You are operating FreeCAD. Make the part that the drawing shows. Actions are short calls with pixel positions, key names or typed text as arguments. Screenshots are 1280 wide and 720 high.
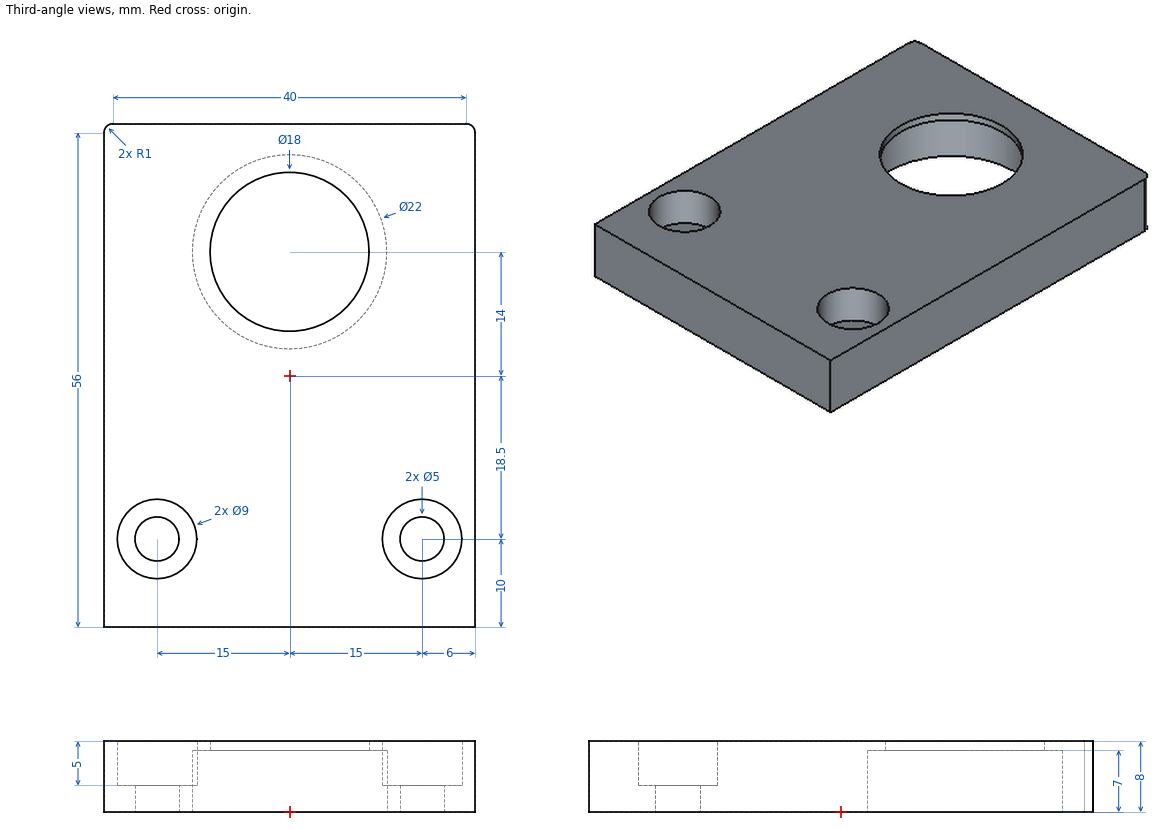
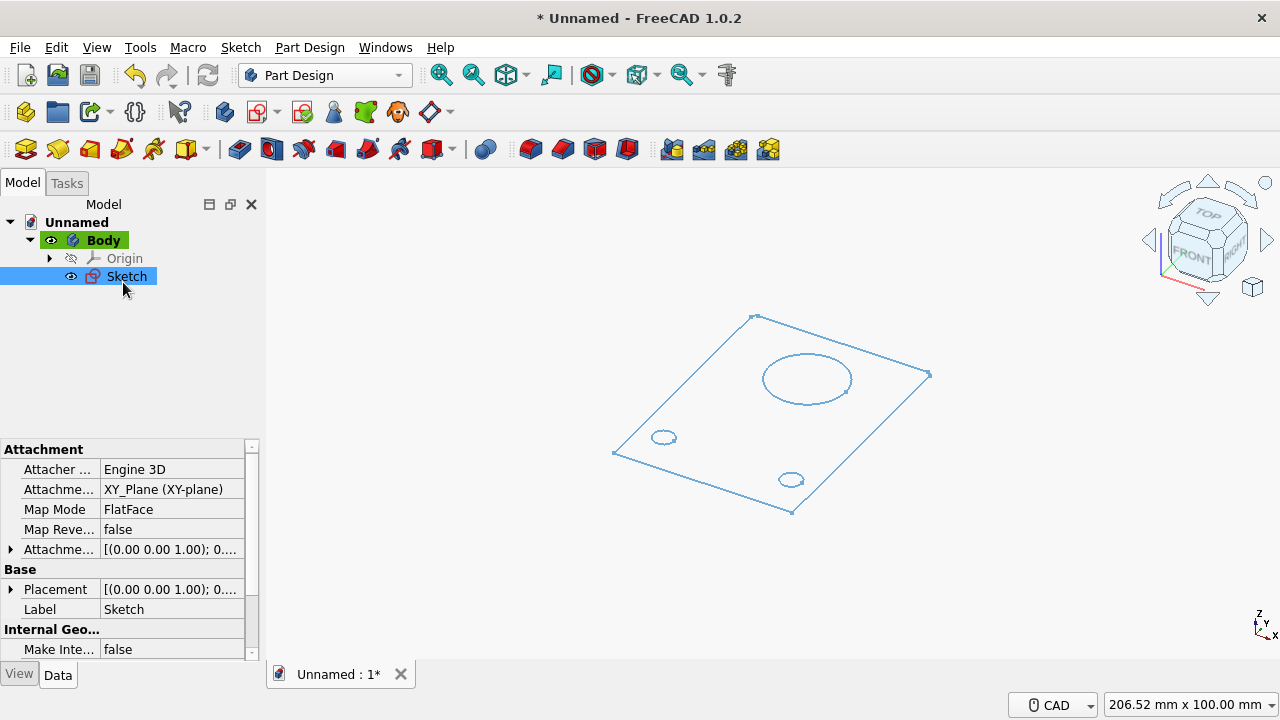
click(26, 150)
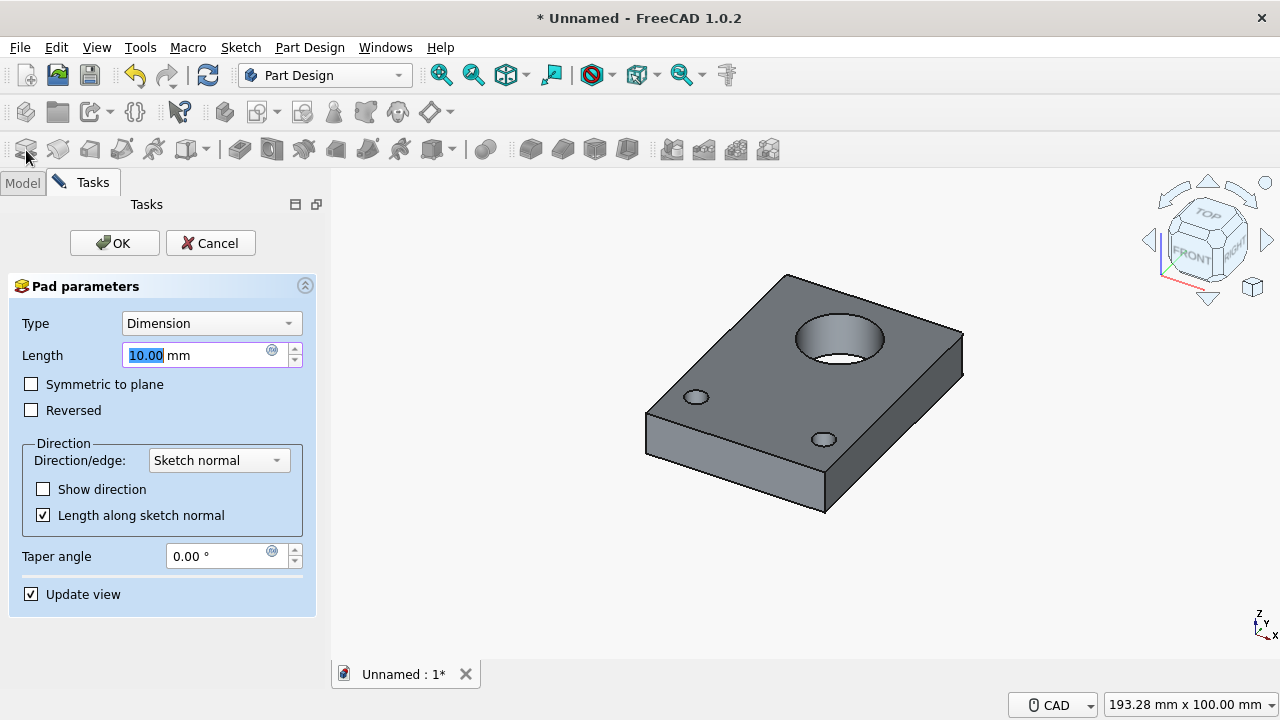
text(8)
key(Tab)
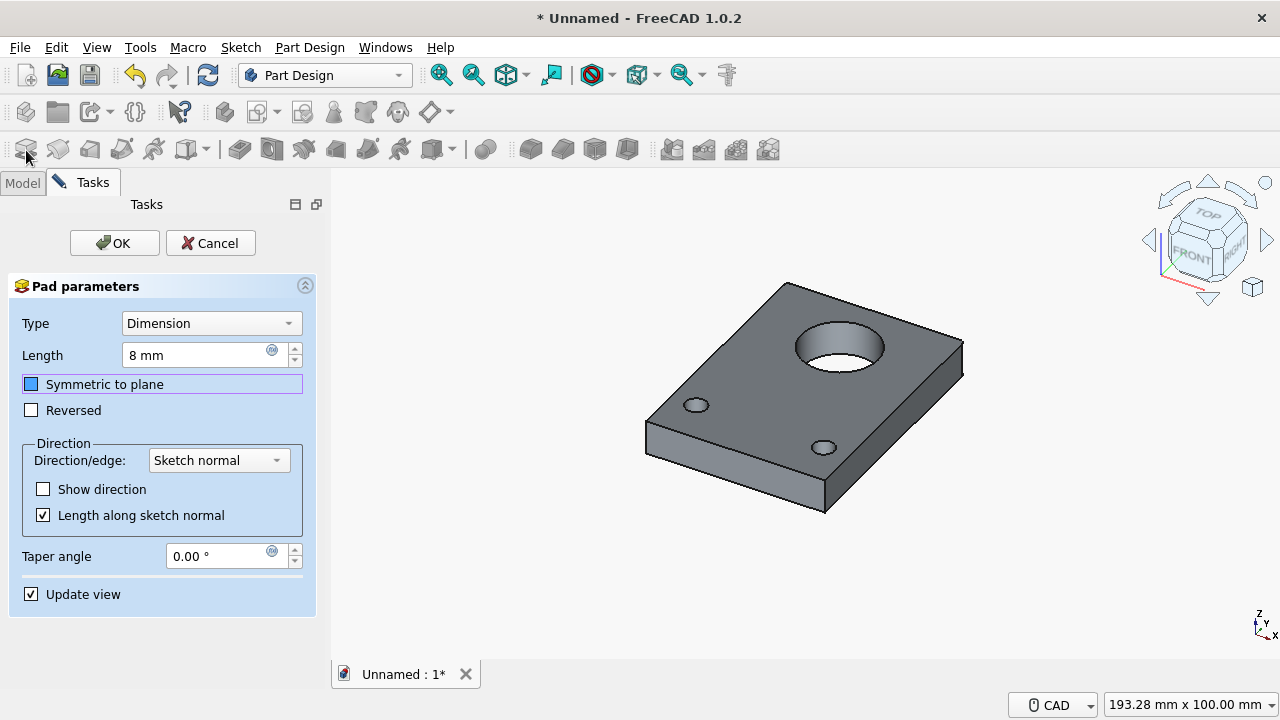
click(115, 243)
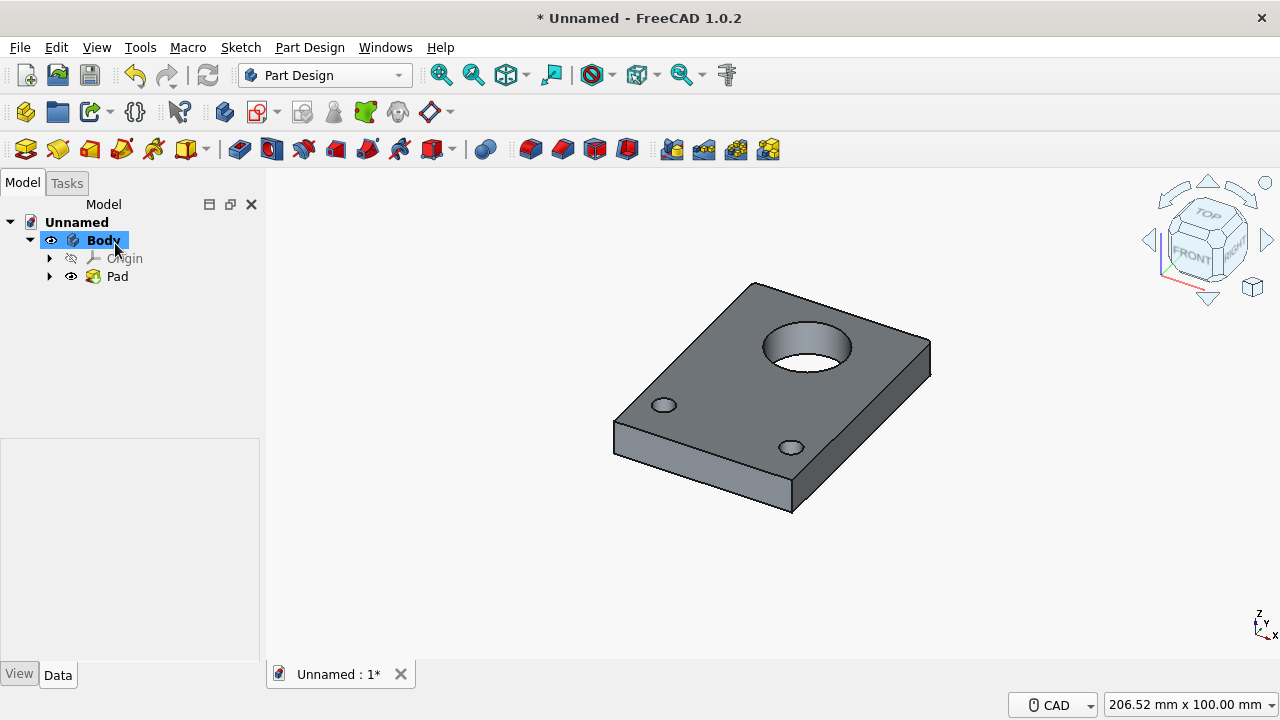
click(753, 400)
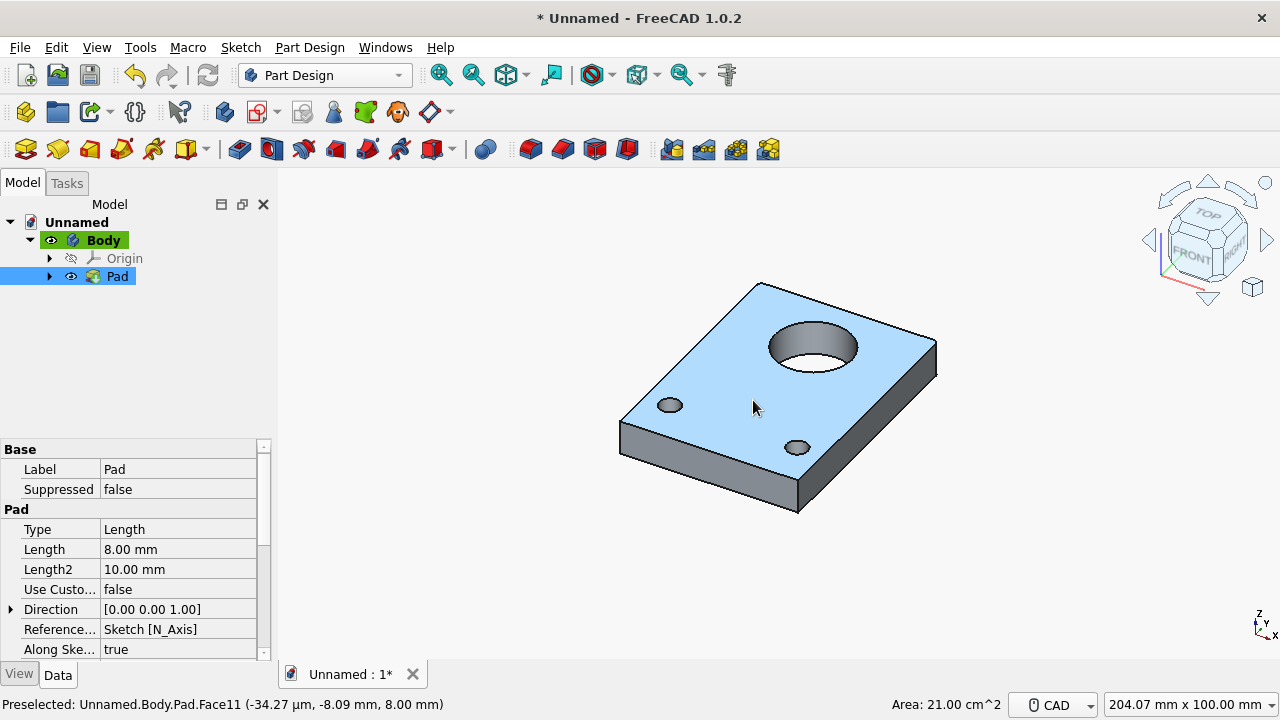
click(258, 112)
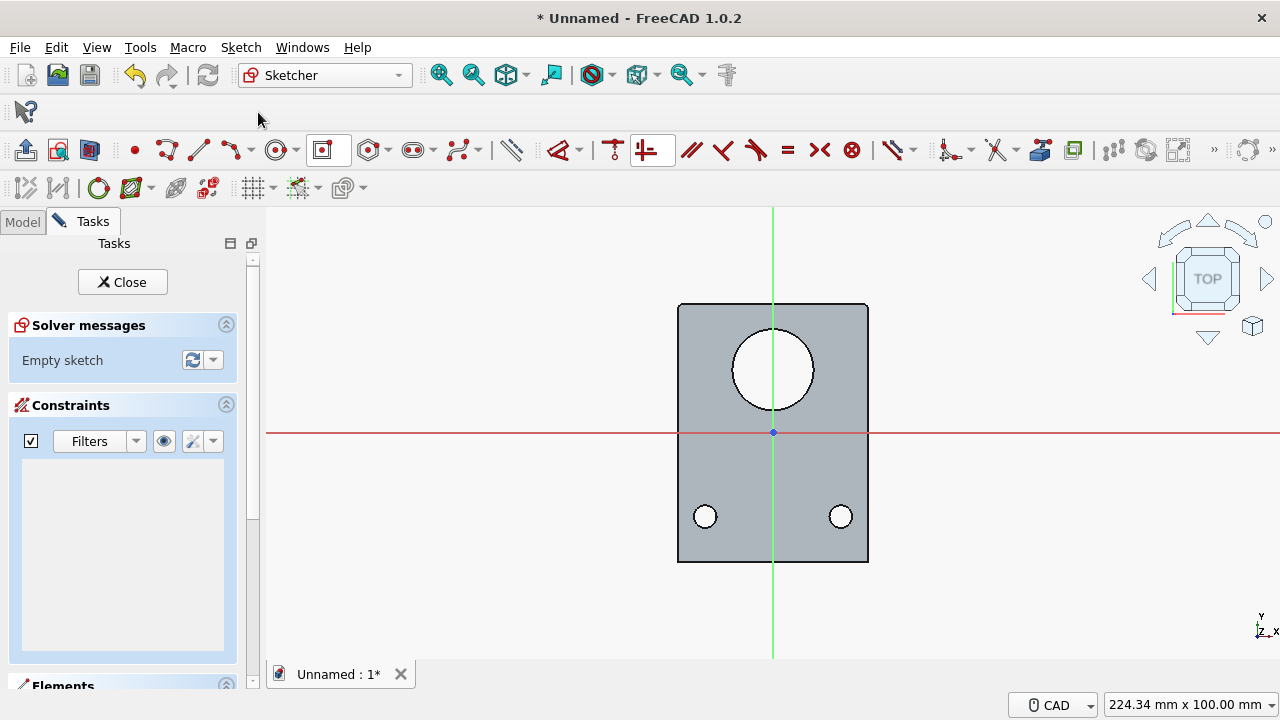
scroll(813, 515, up, 5)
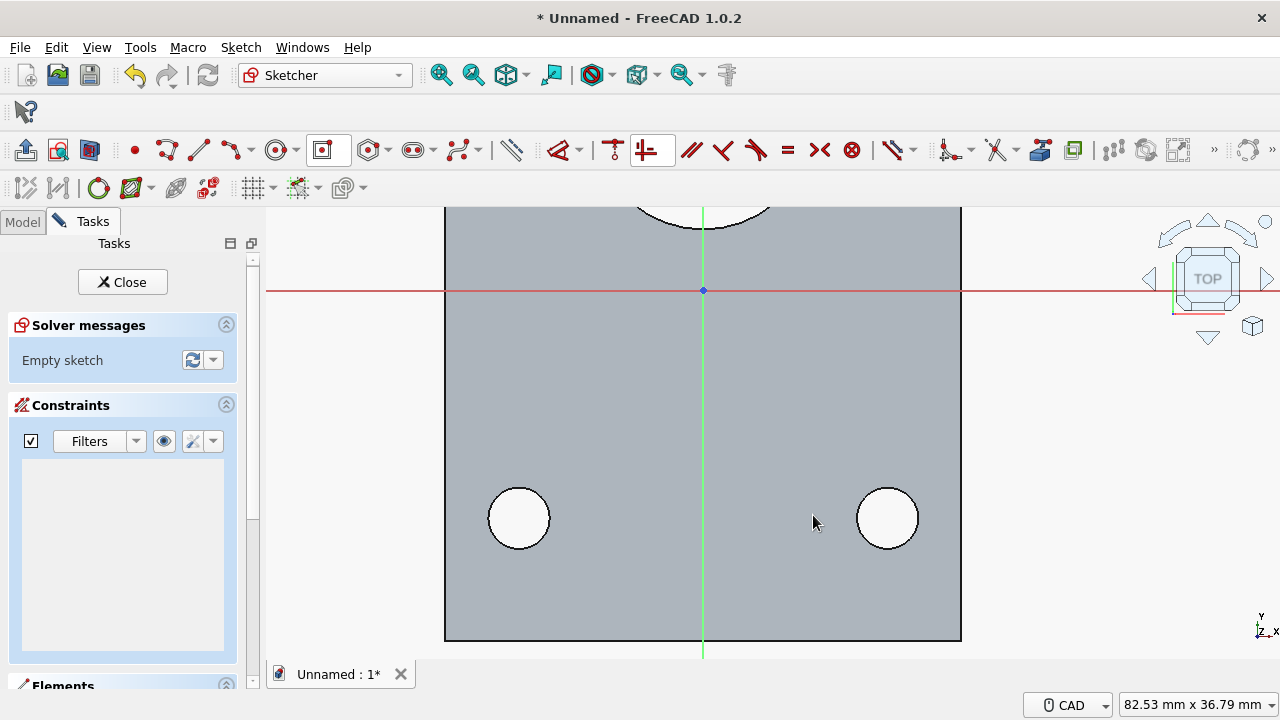
click(276, 150)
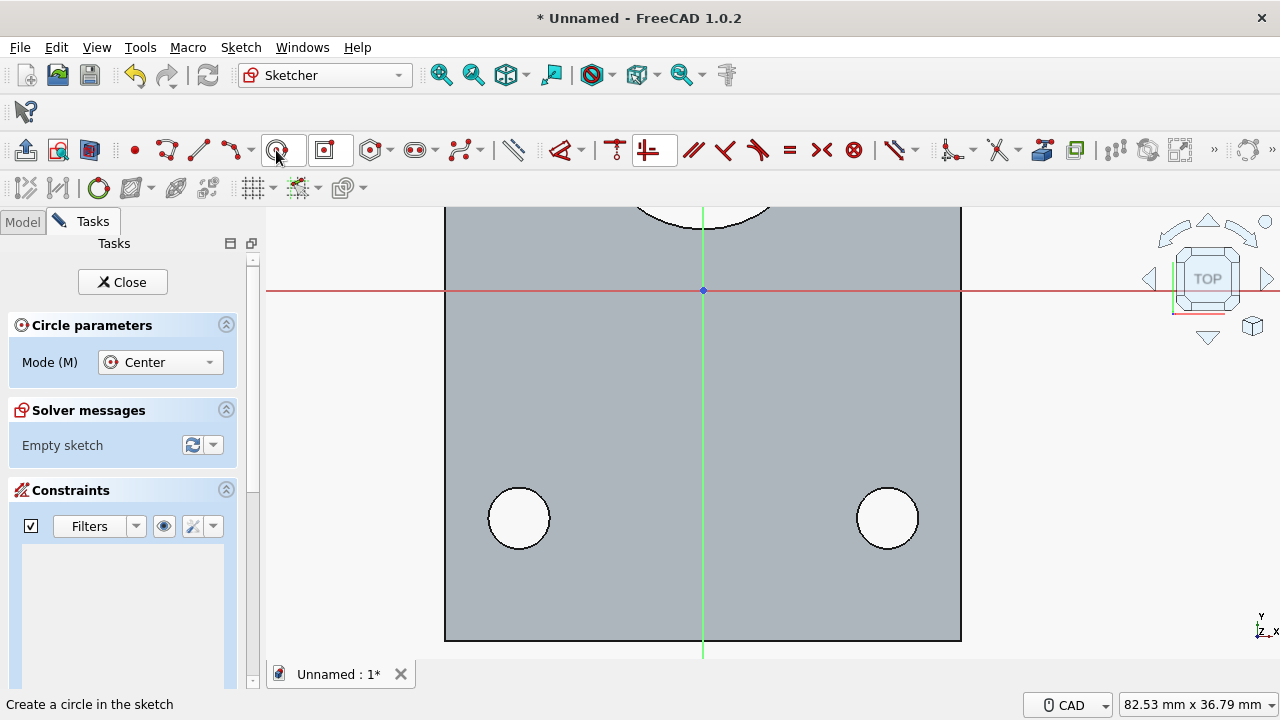
click(519, 518)
click(558, 479)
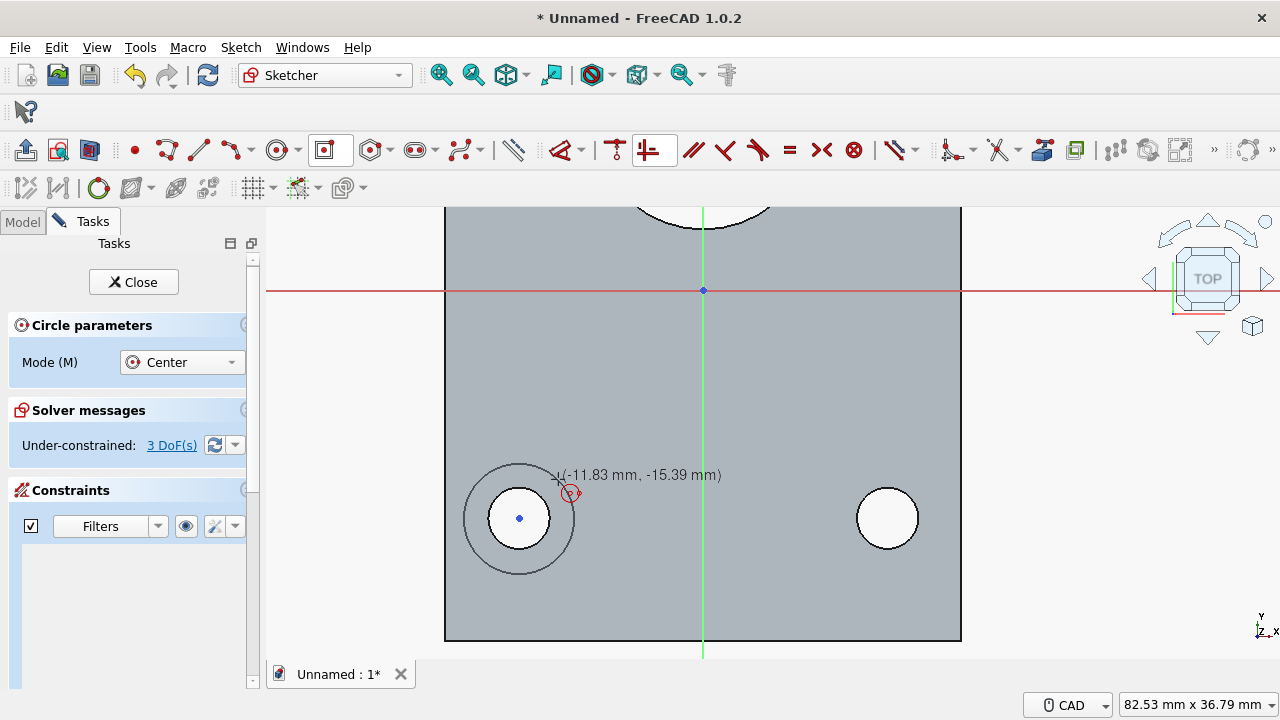
click(888, 518)
click(927, 479)
key(Escape)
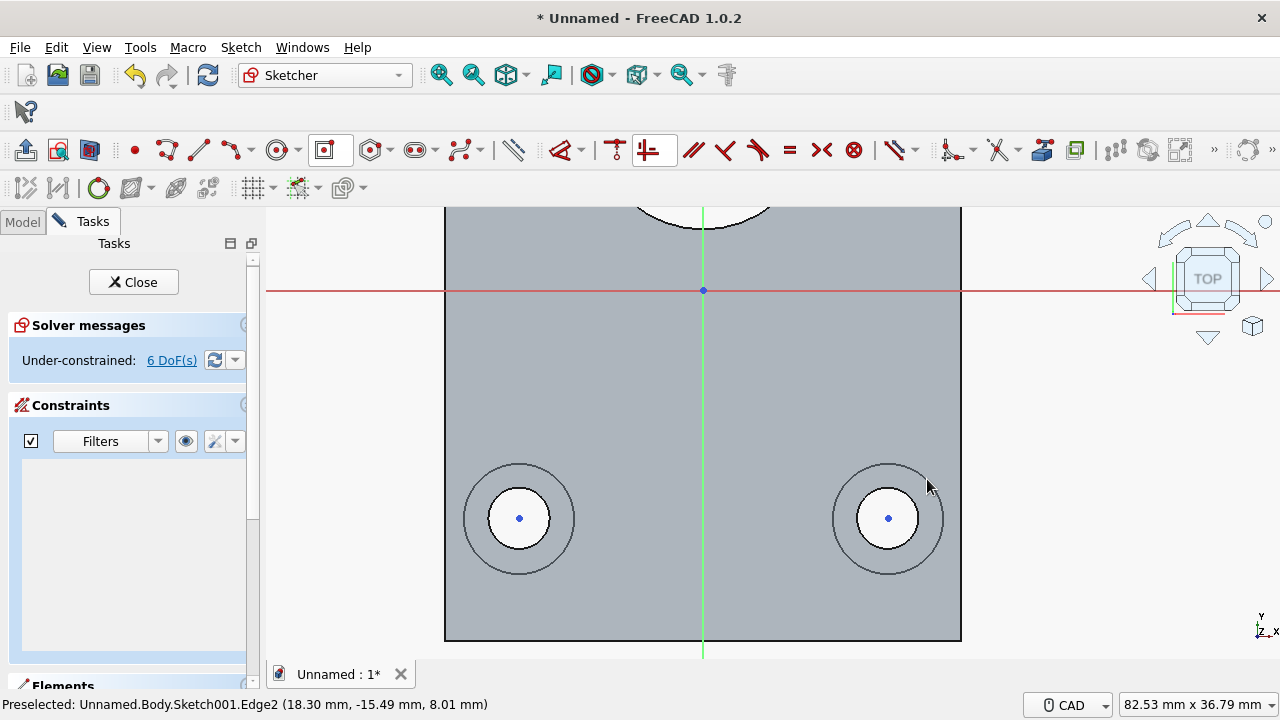
click(558, 480)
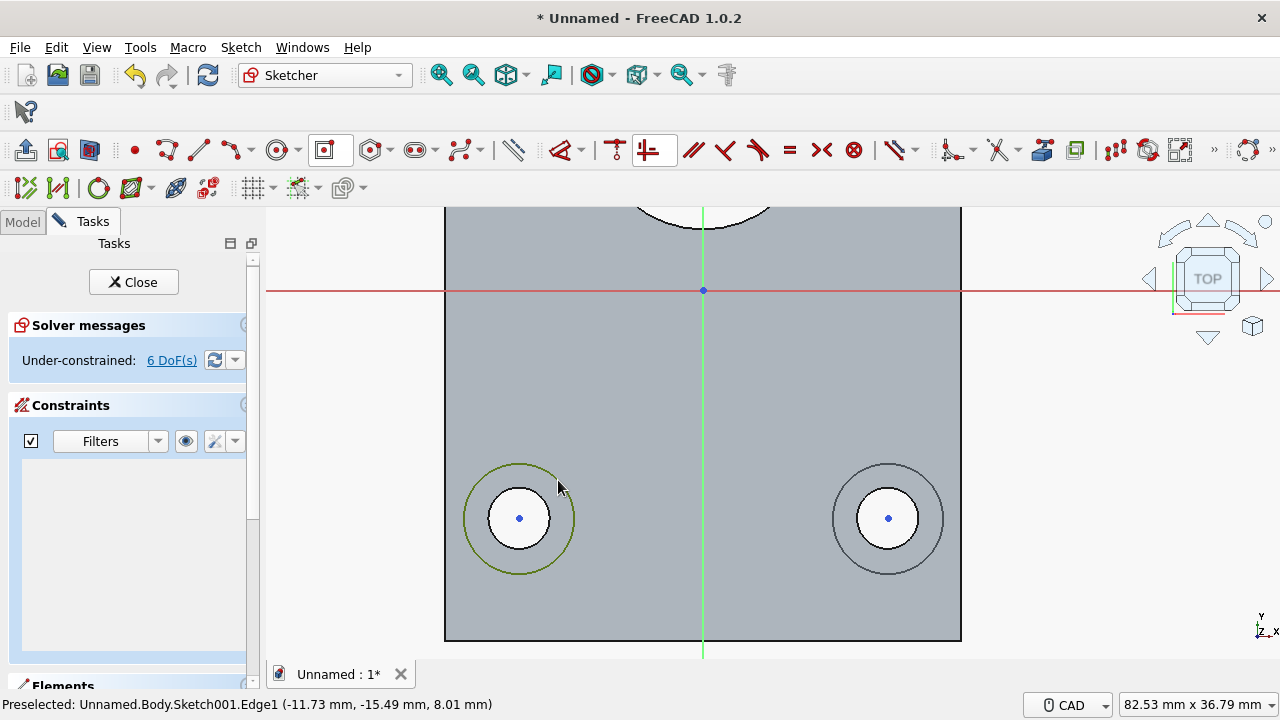
click(927, 480)